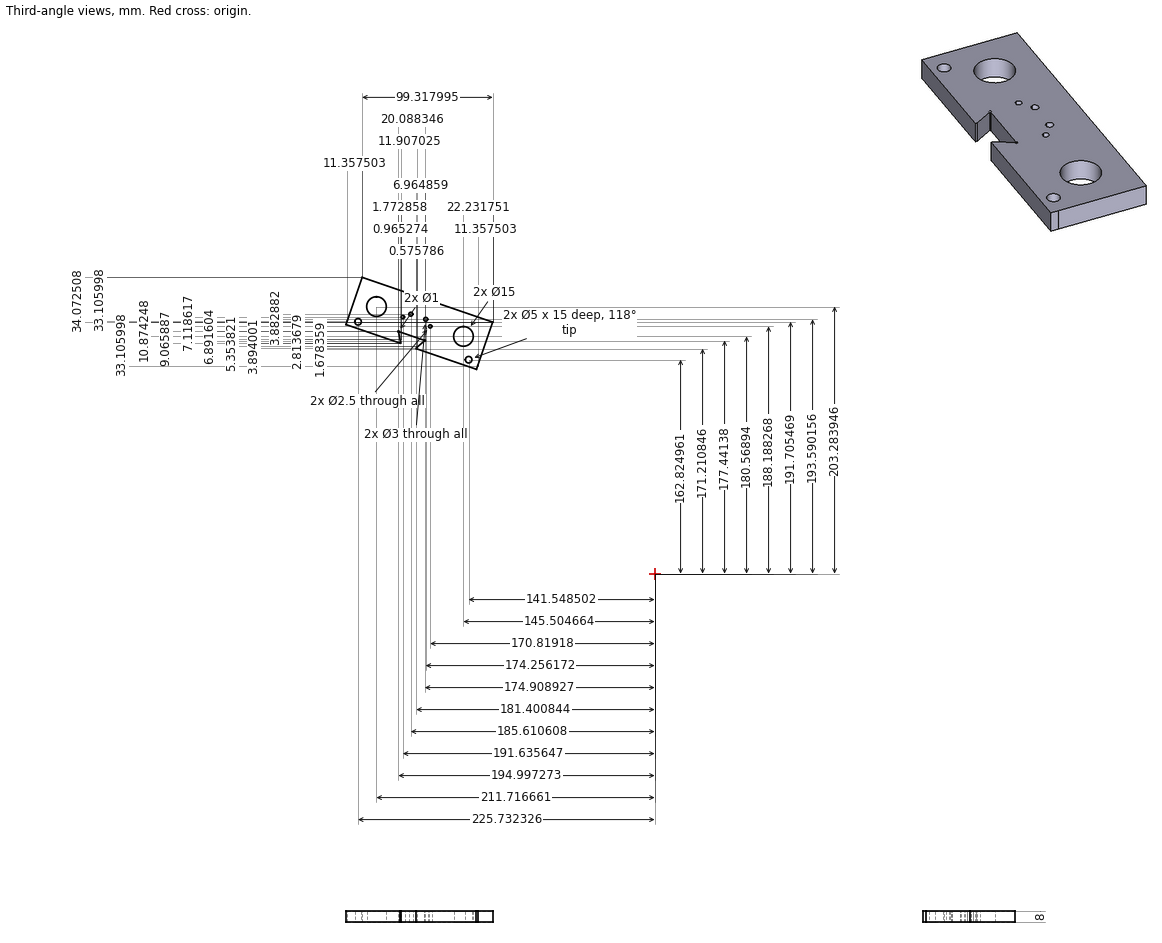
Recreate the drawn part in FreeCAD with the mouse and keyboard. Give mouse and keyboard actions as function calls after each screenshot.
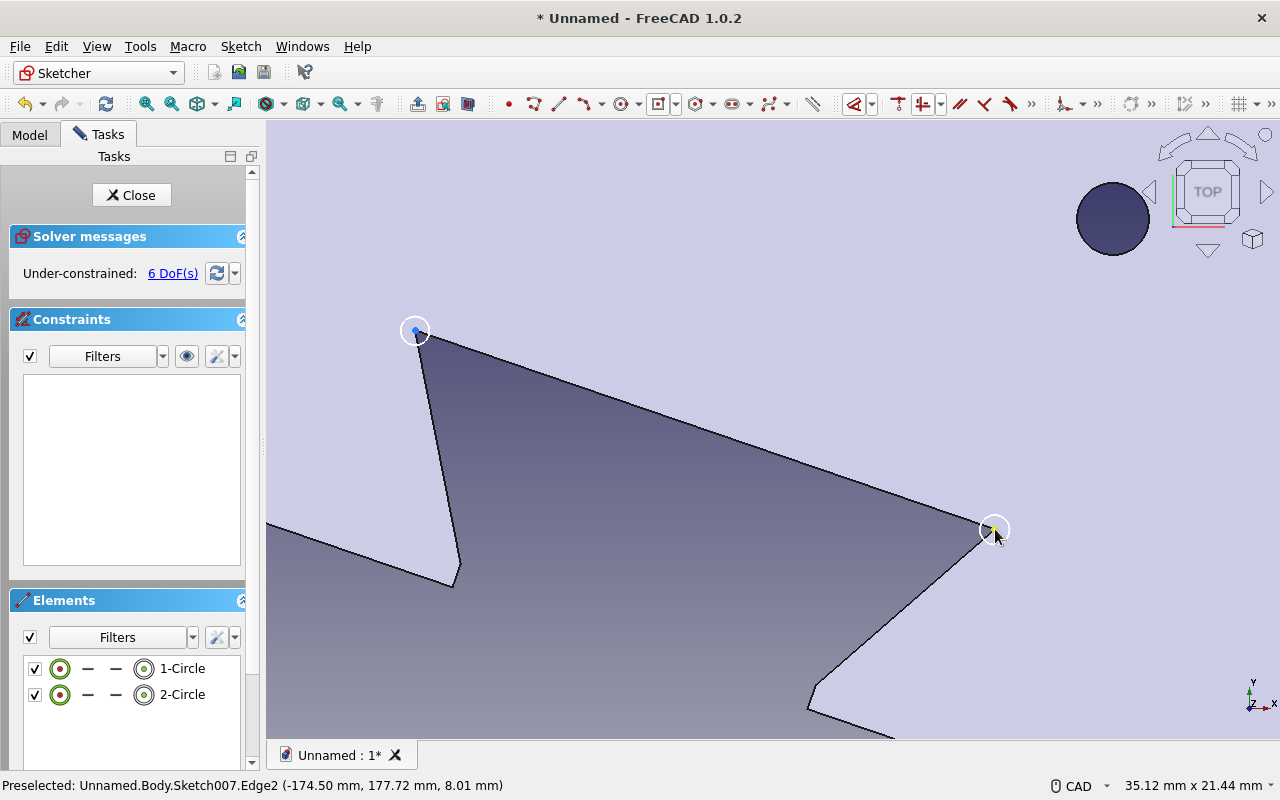
click(425, 321)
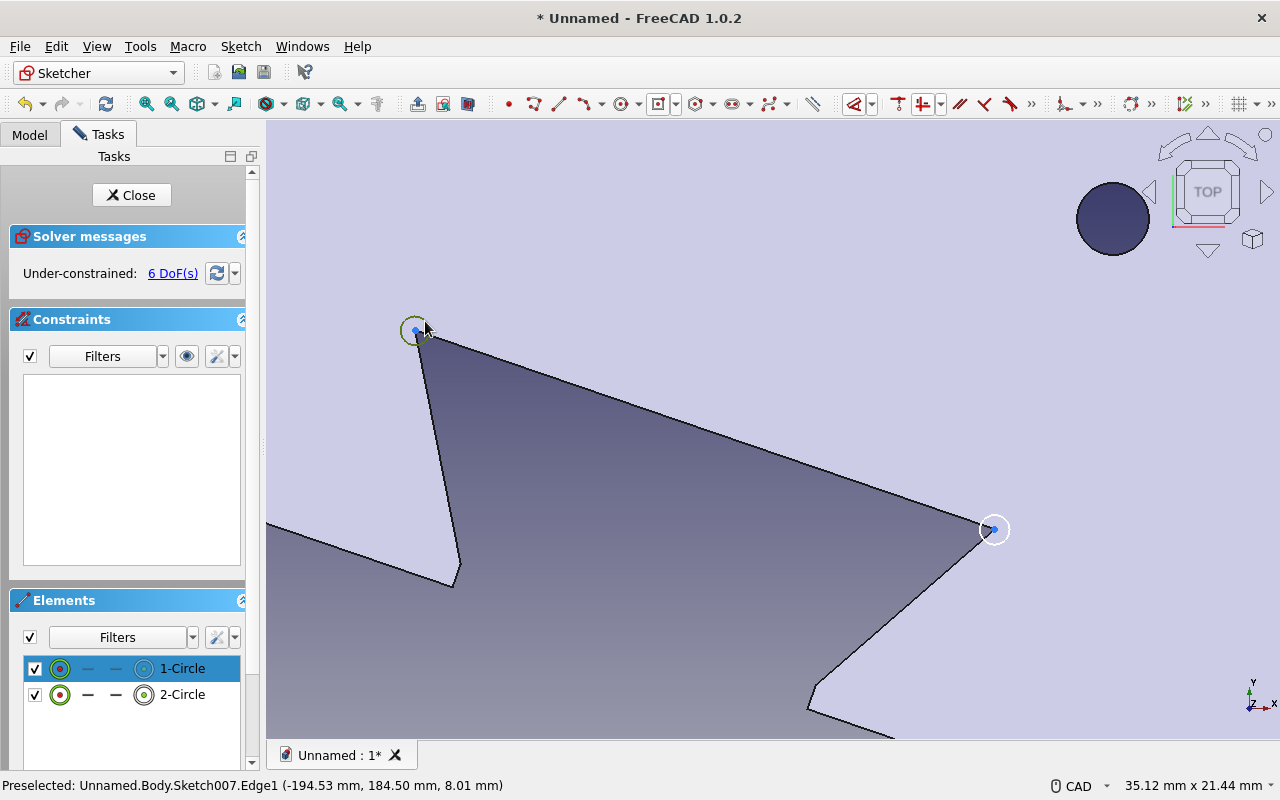
click(1005, 519)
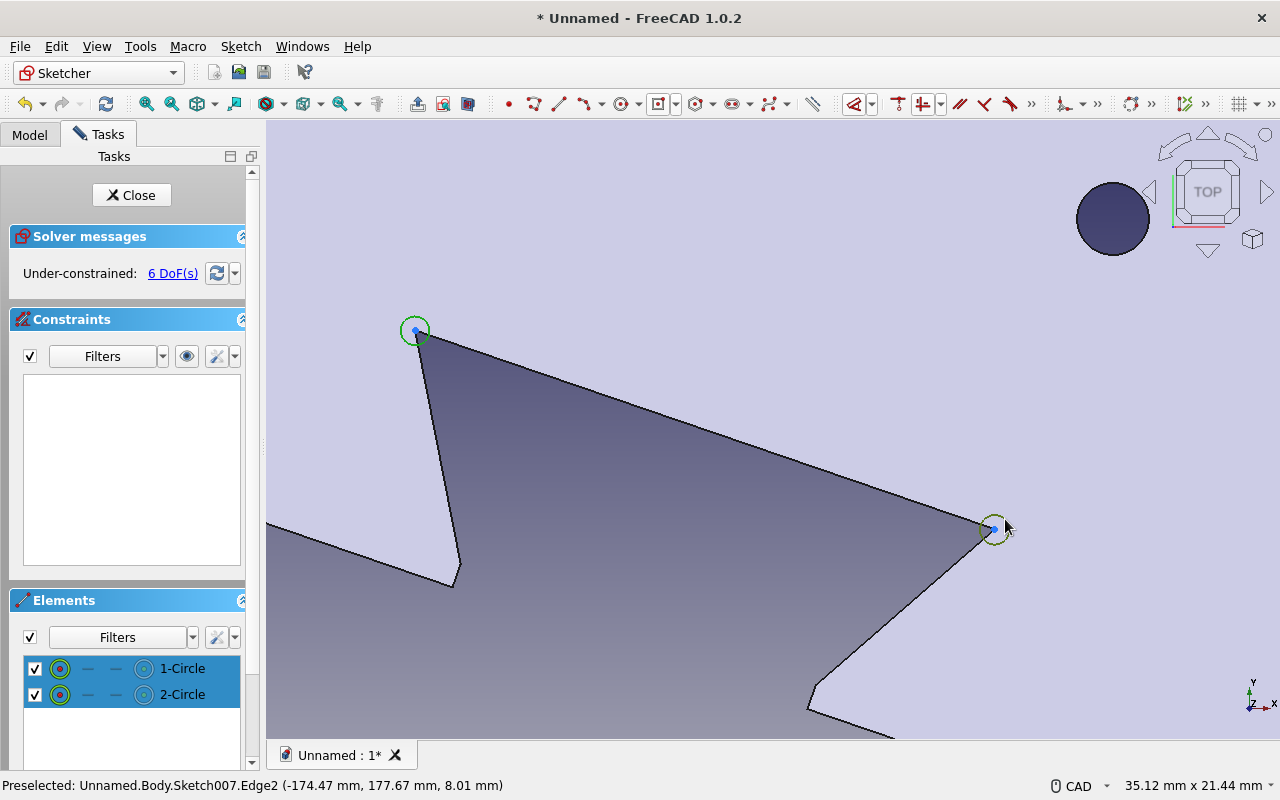
key(e)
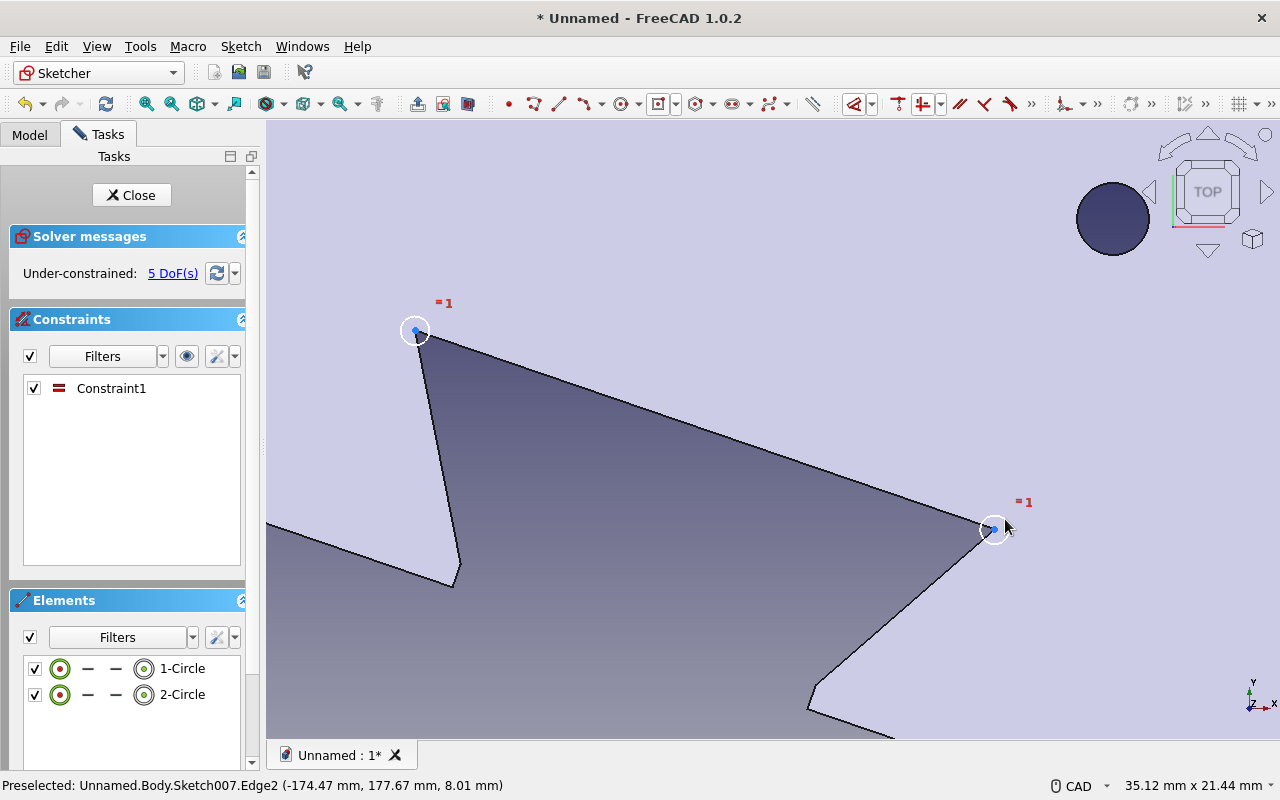
scroll(425, 321, up, 2)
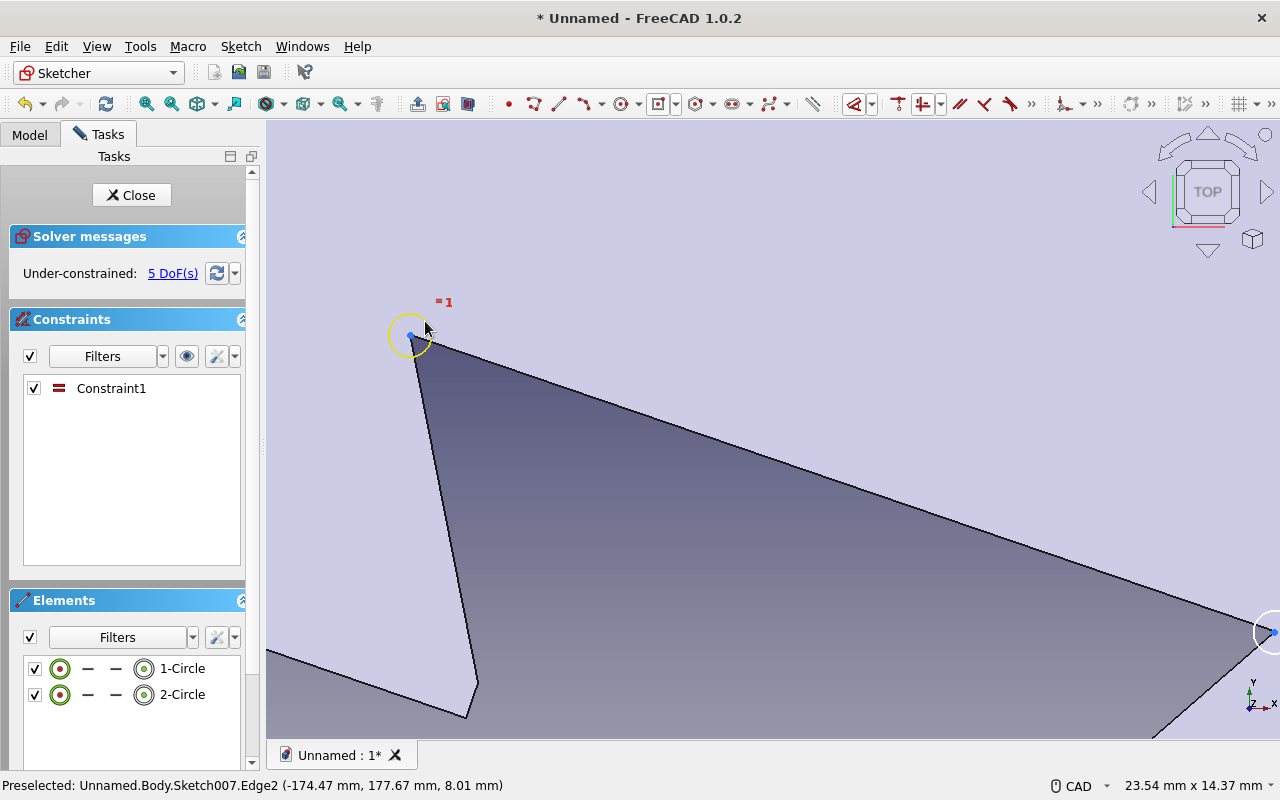
click(425, 320)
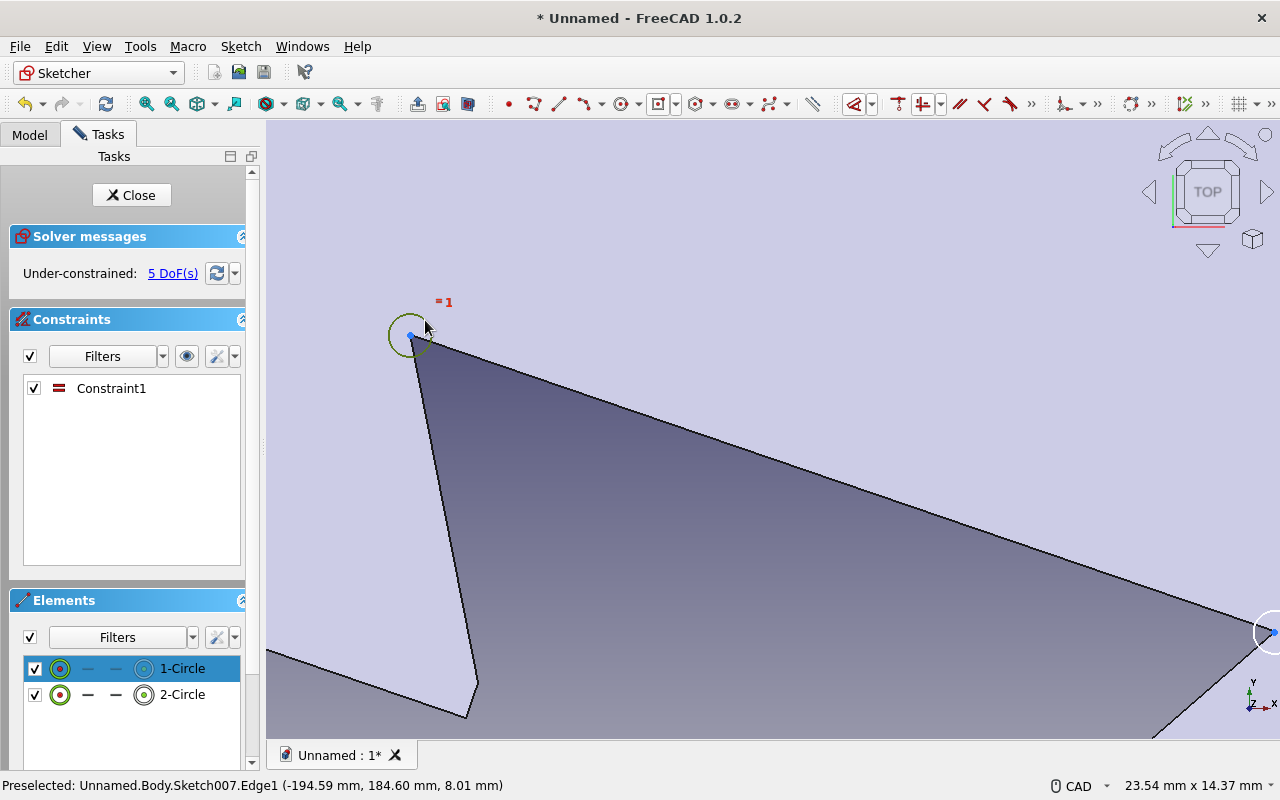
key(k)
key(o)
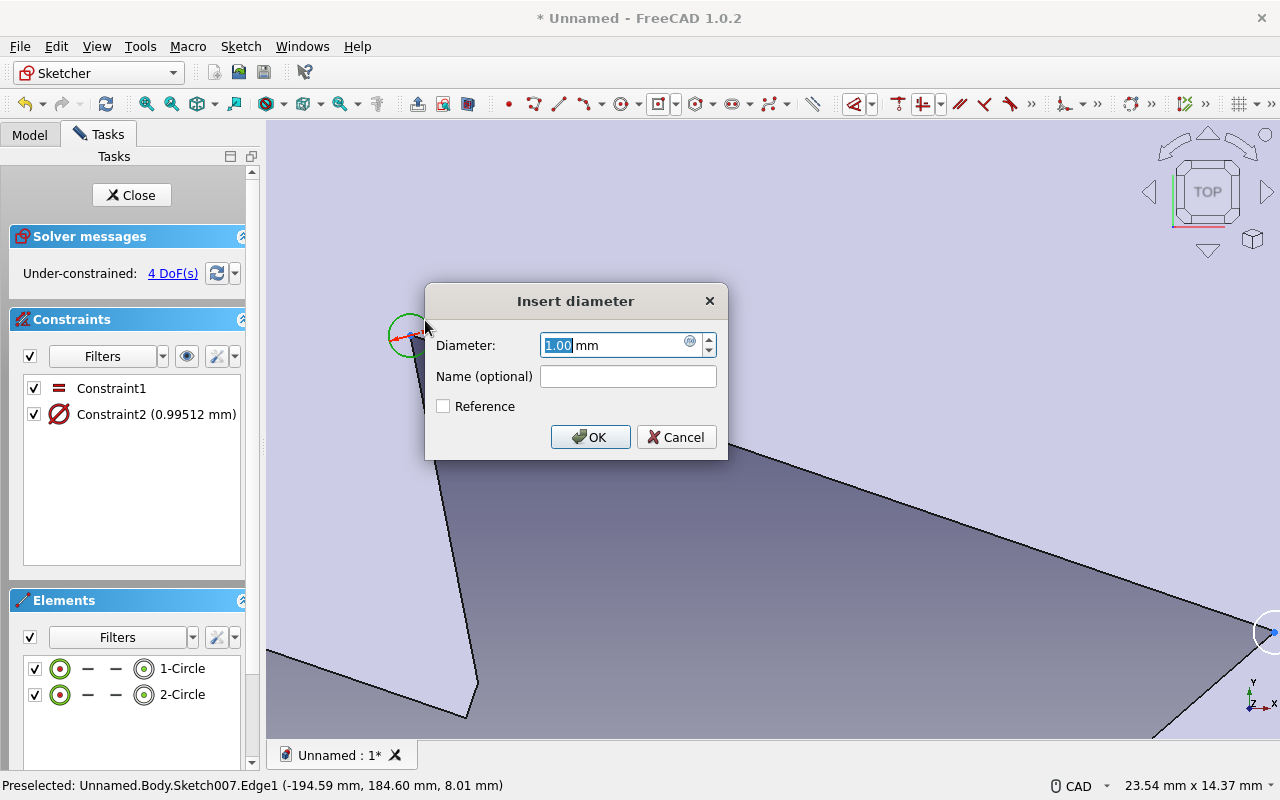
text(1)
key(Return)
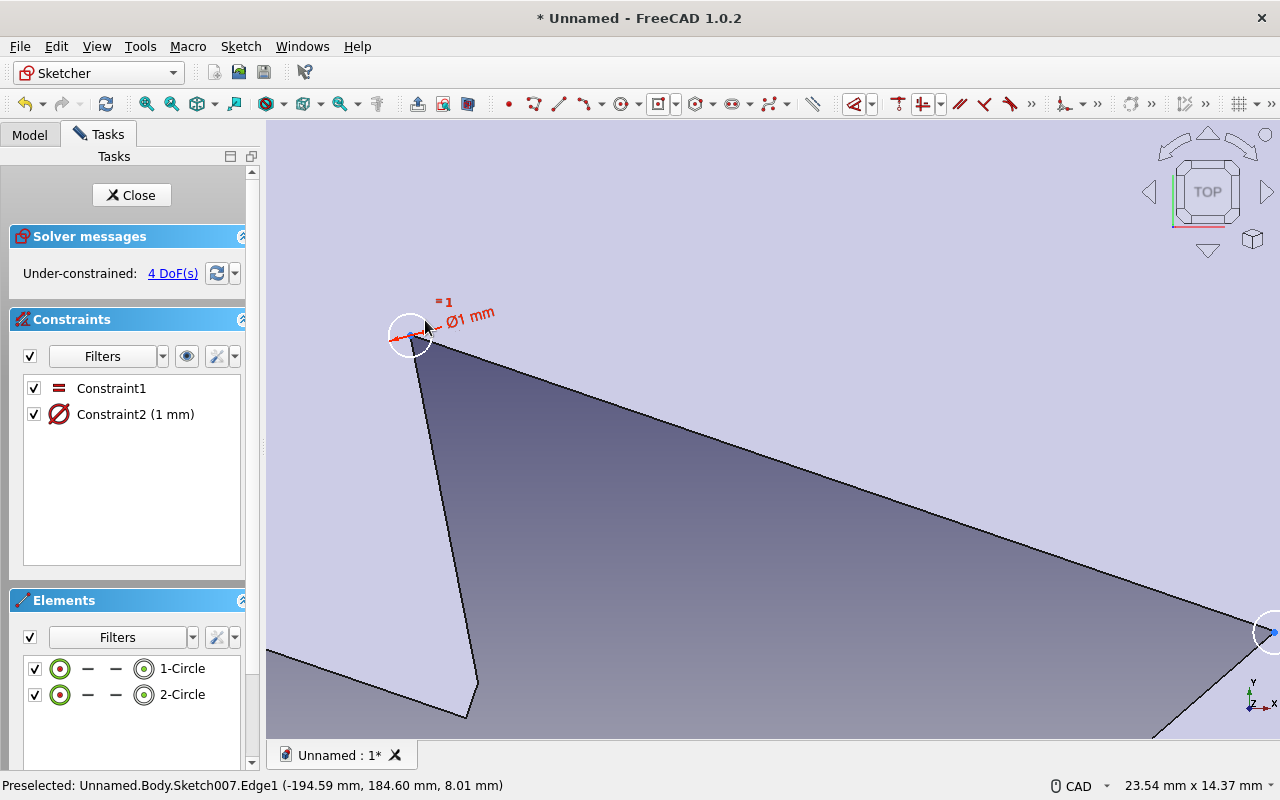
scroll(424, 321, down, 2)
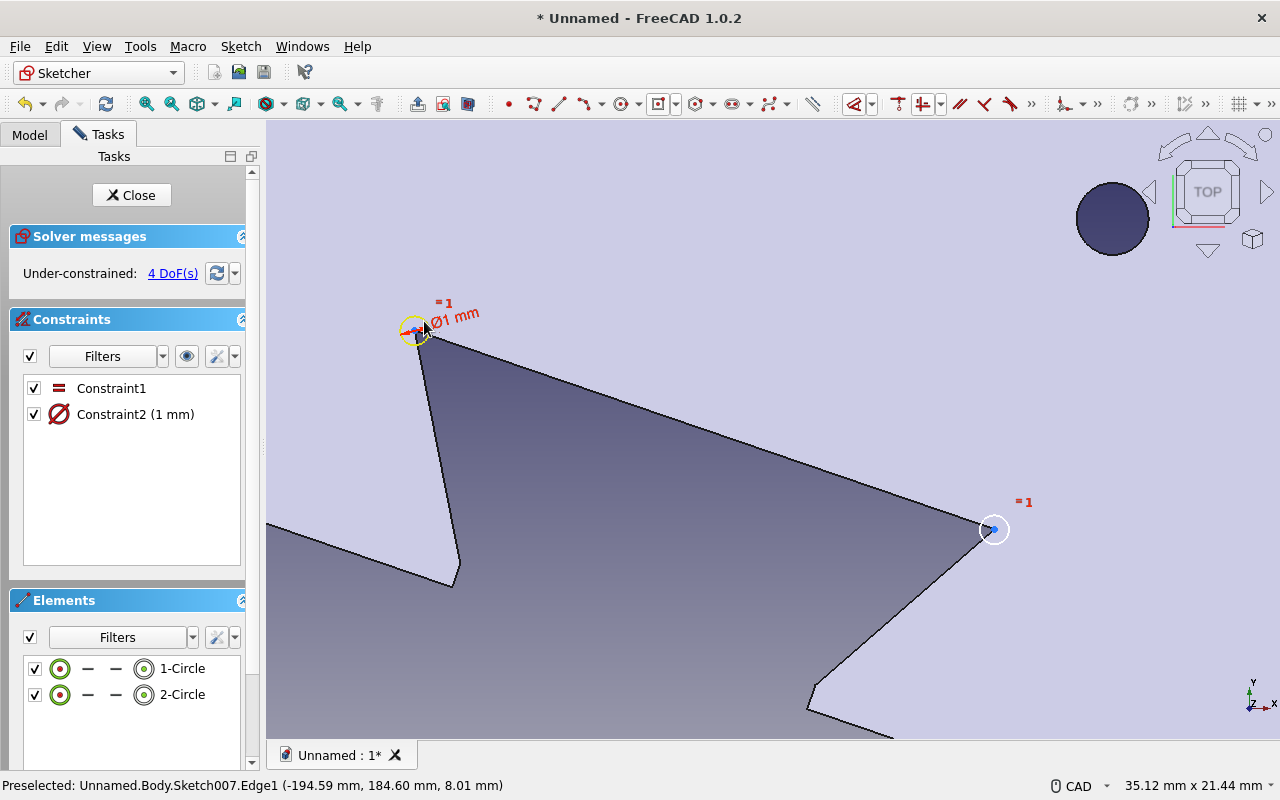
click(994, 530)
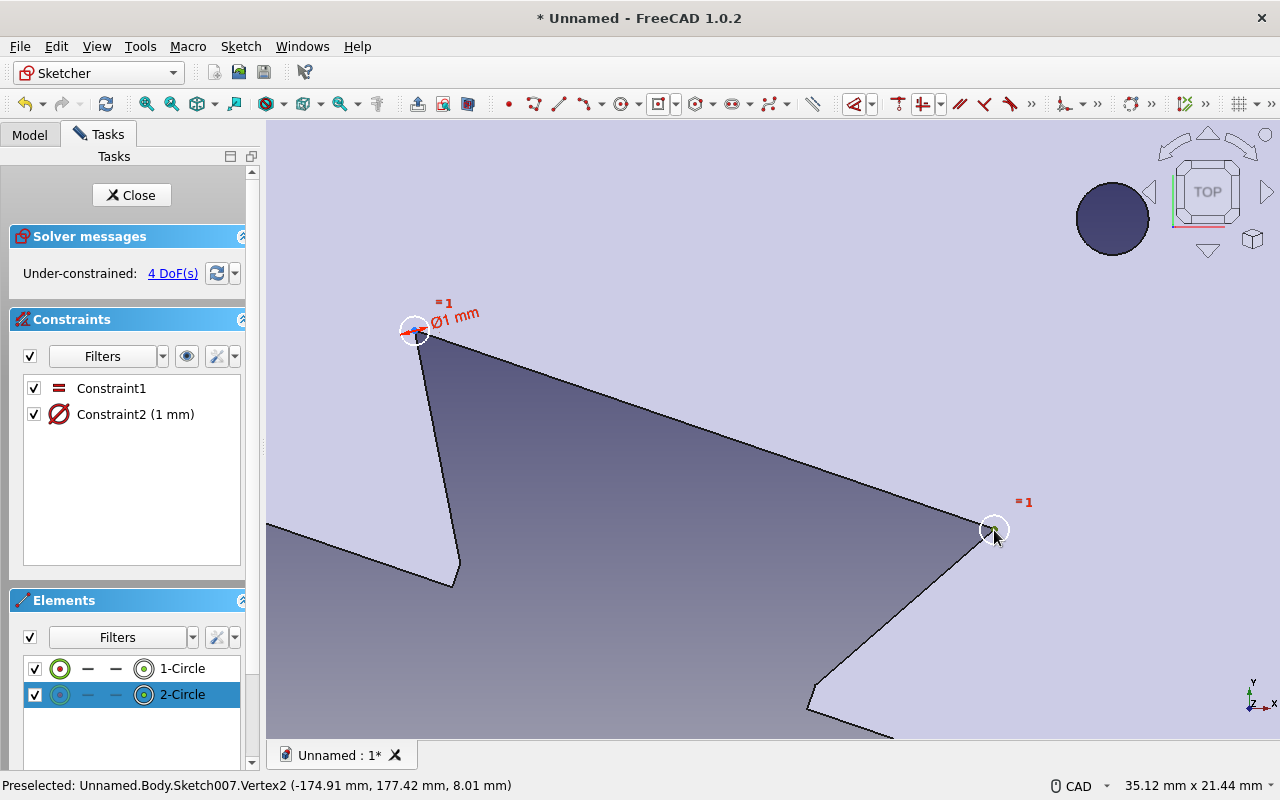
click(872, 104)